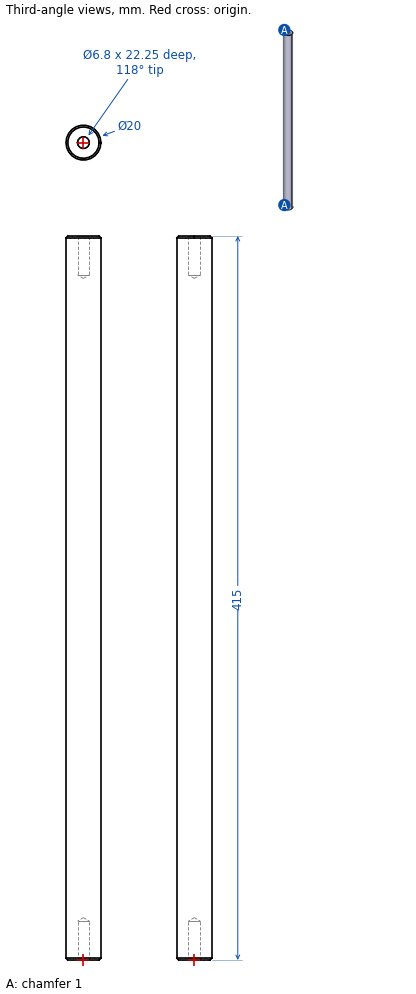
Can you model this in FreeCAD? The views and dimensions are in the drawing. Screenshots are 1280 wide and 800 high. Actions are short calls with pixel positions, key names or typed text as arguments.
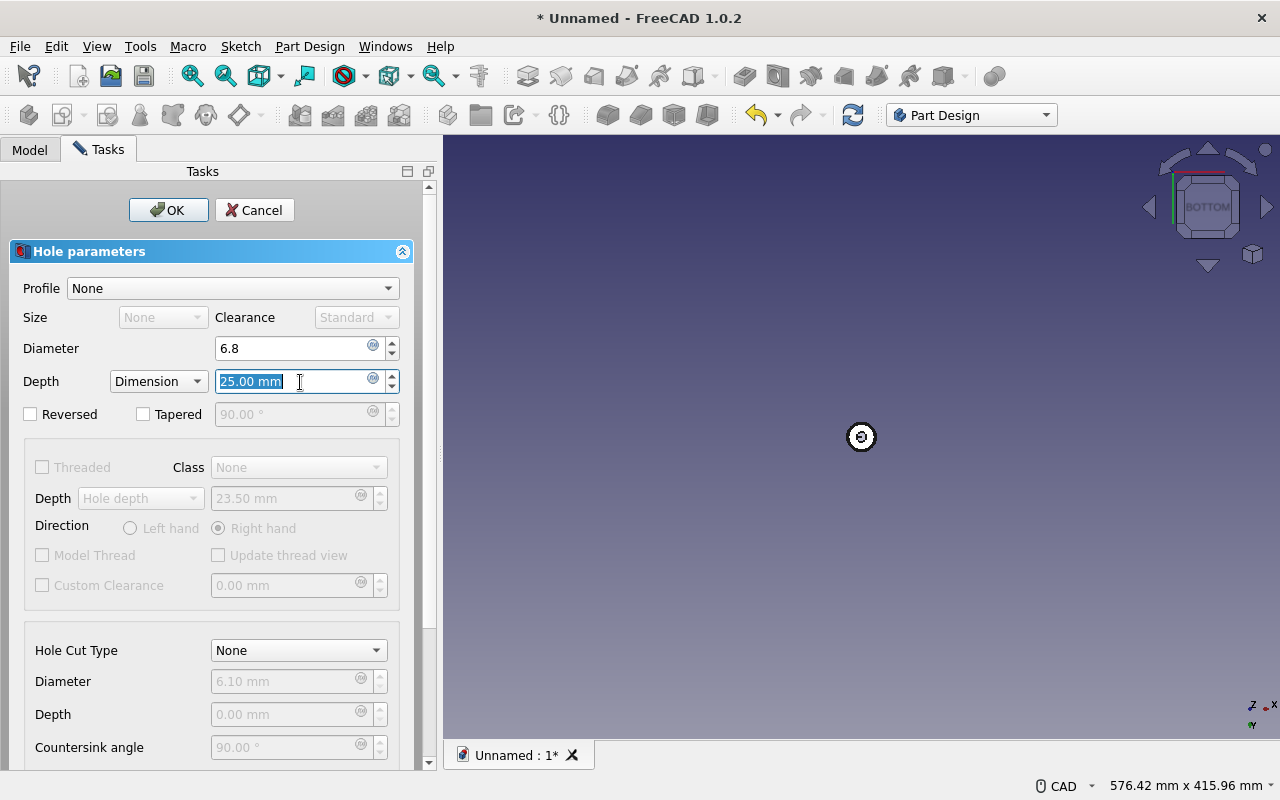
text(22.25)
key(Tab)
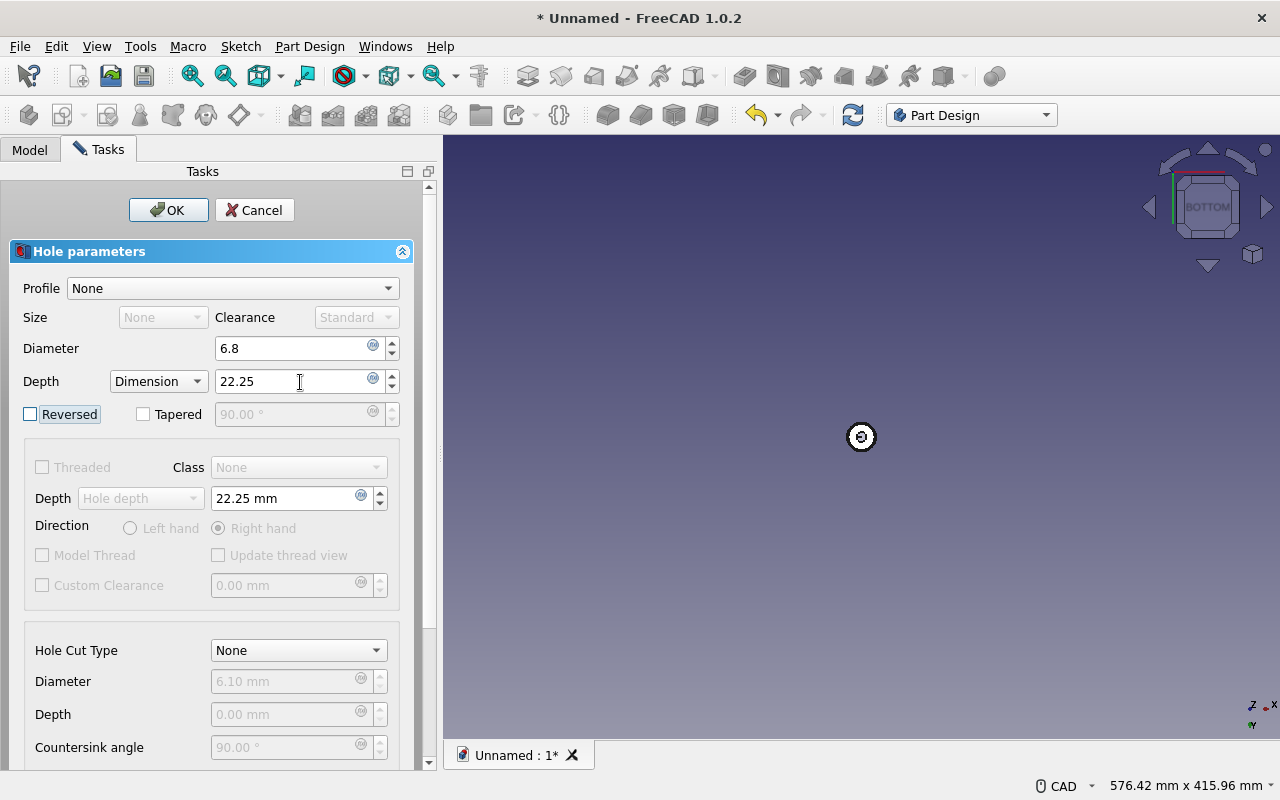
click(169, 210)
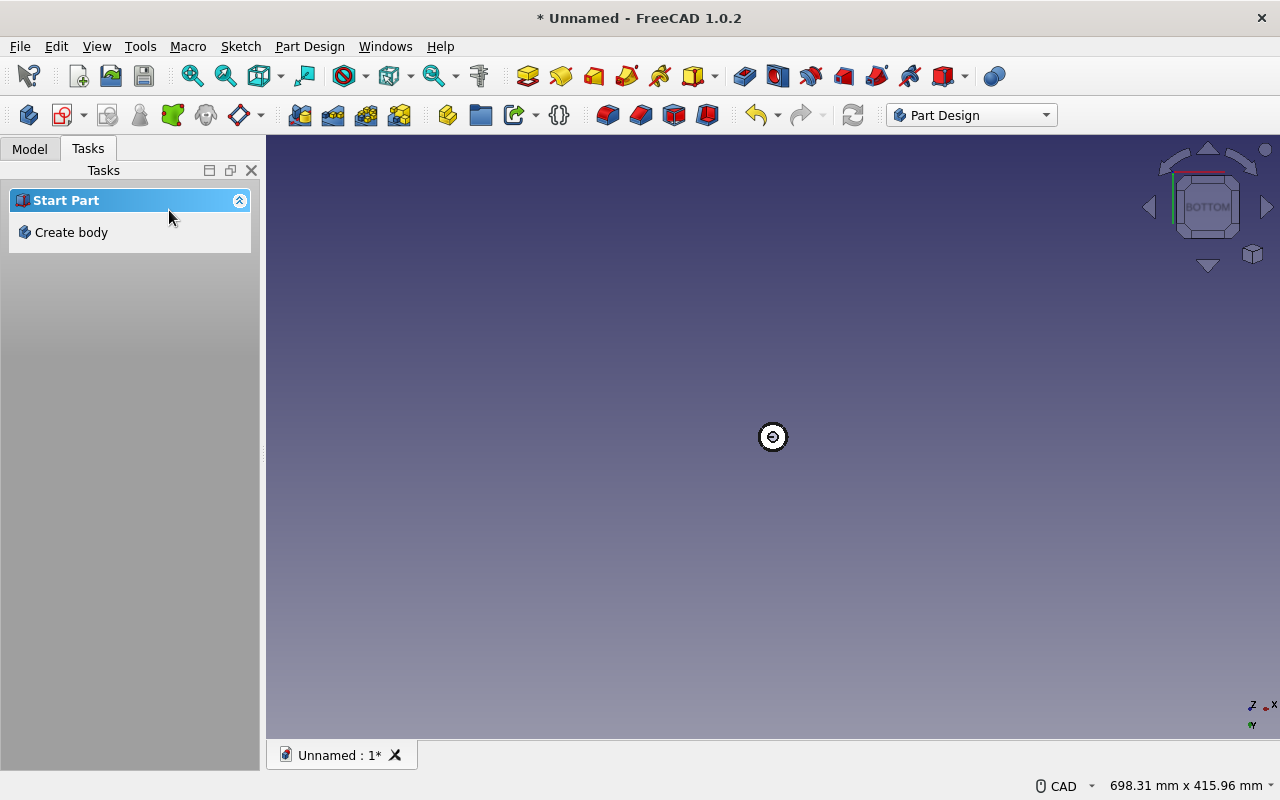
key(0)